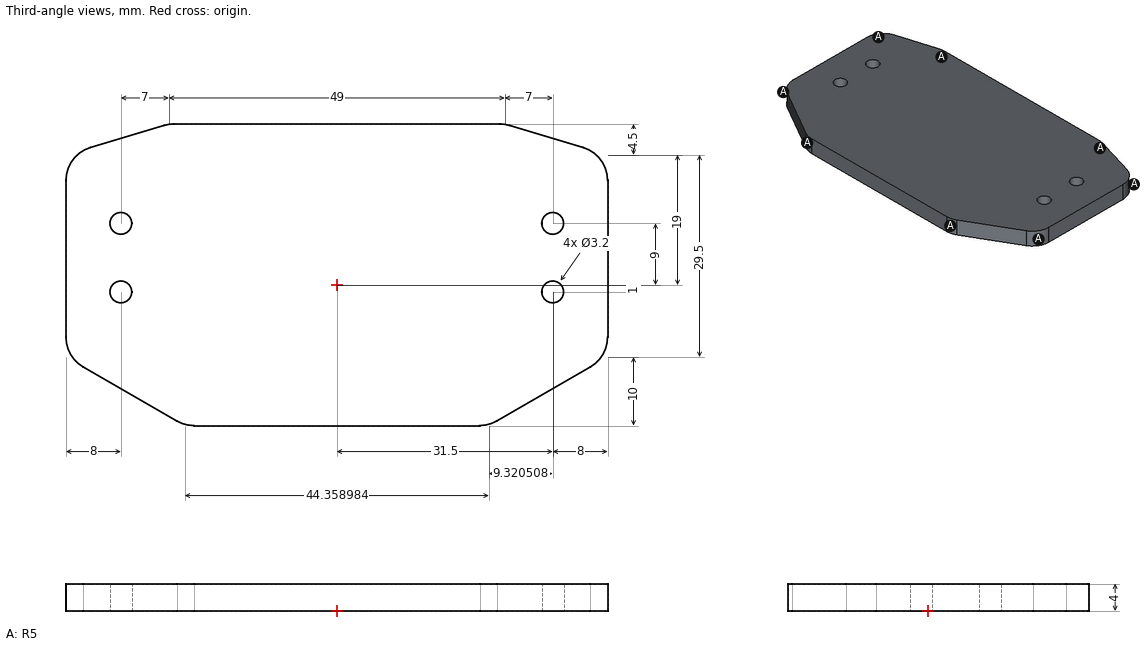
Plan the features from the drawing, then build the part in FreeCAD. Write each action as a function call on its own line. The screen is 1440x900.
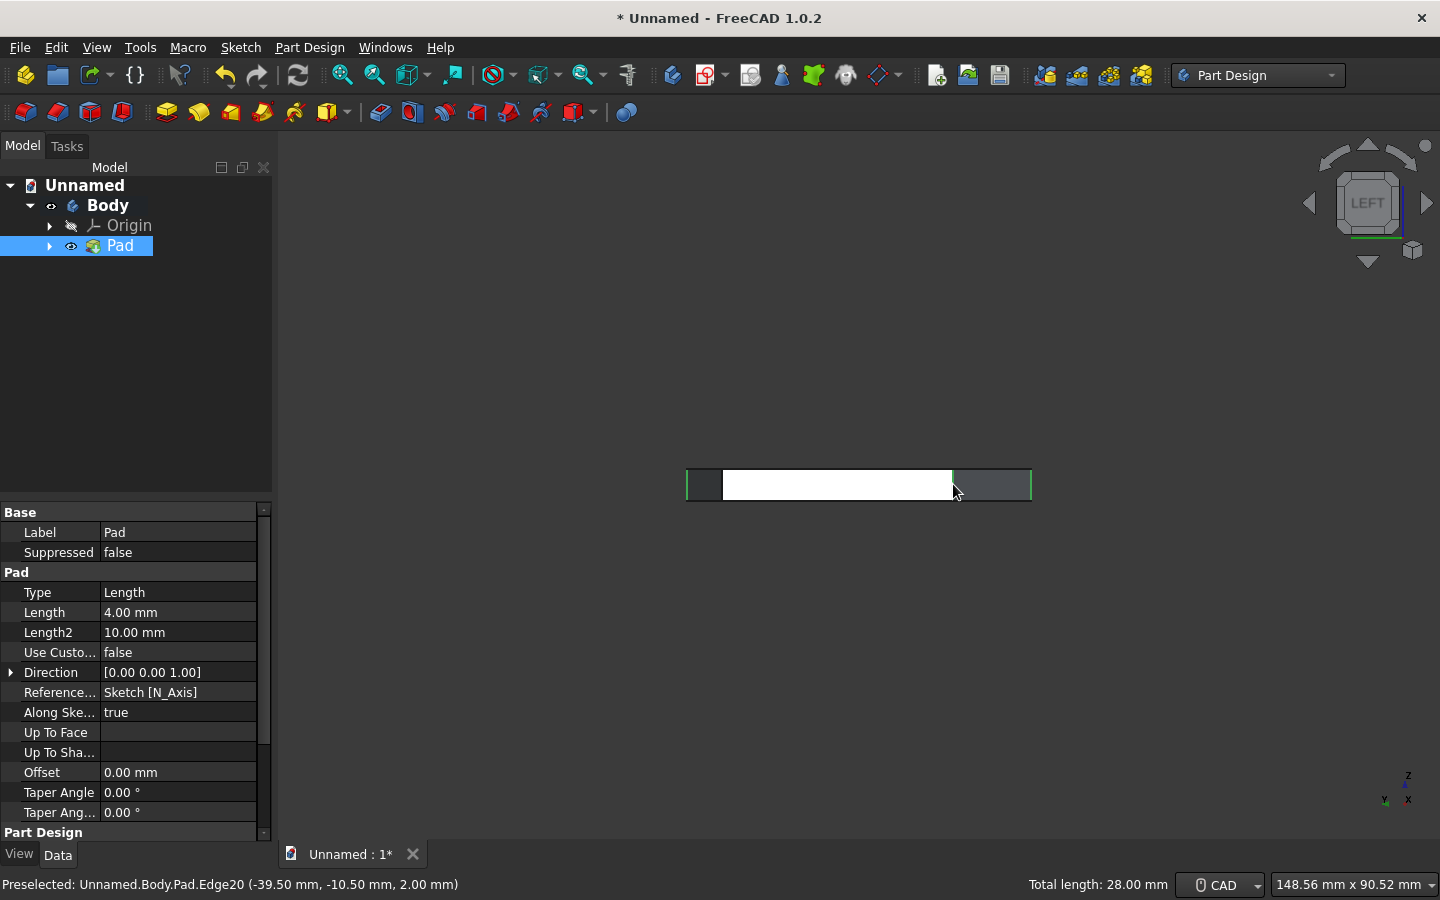
click(722, 484, ctrl)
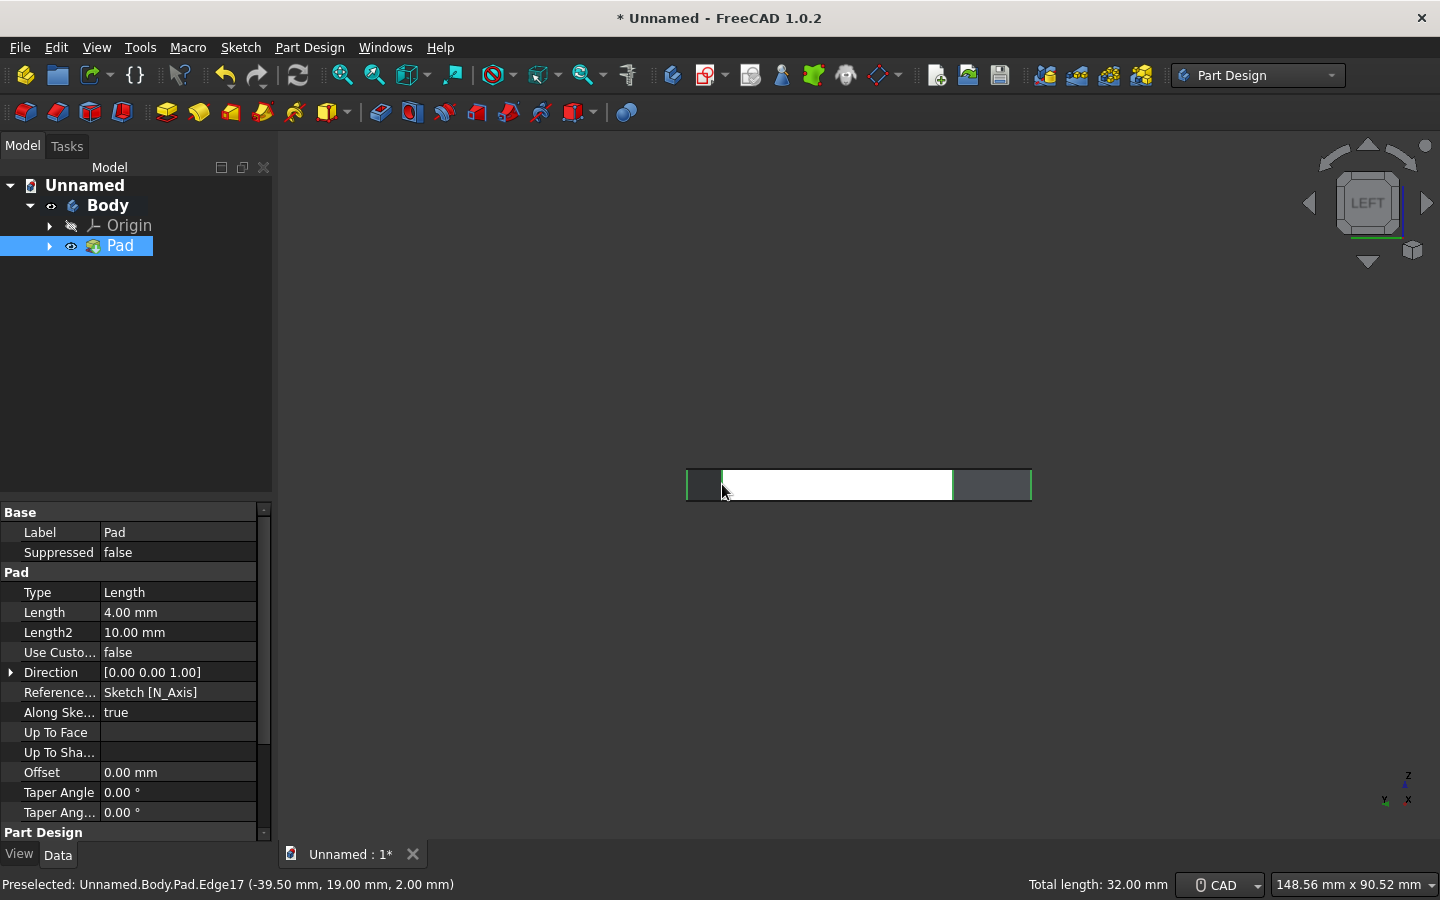
click(26, 112)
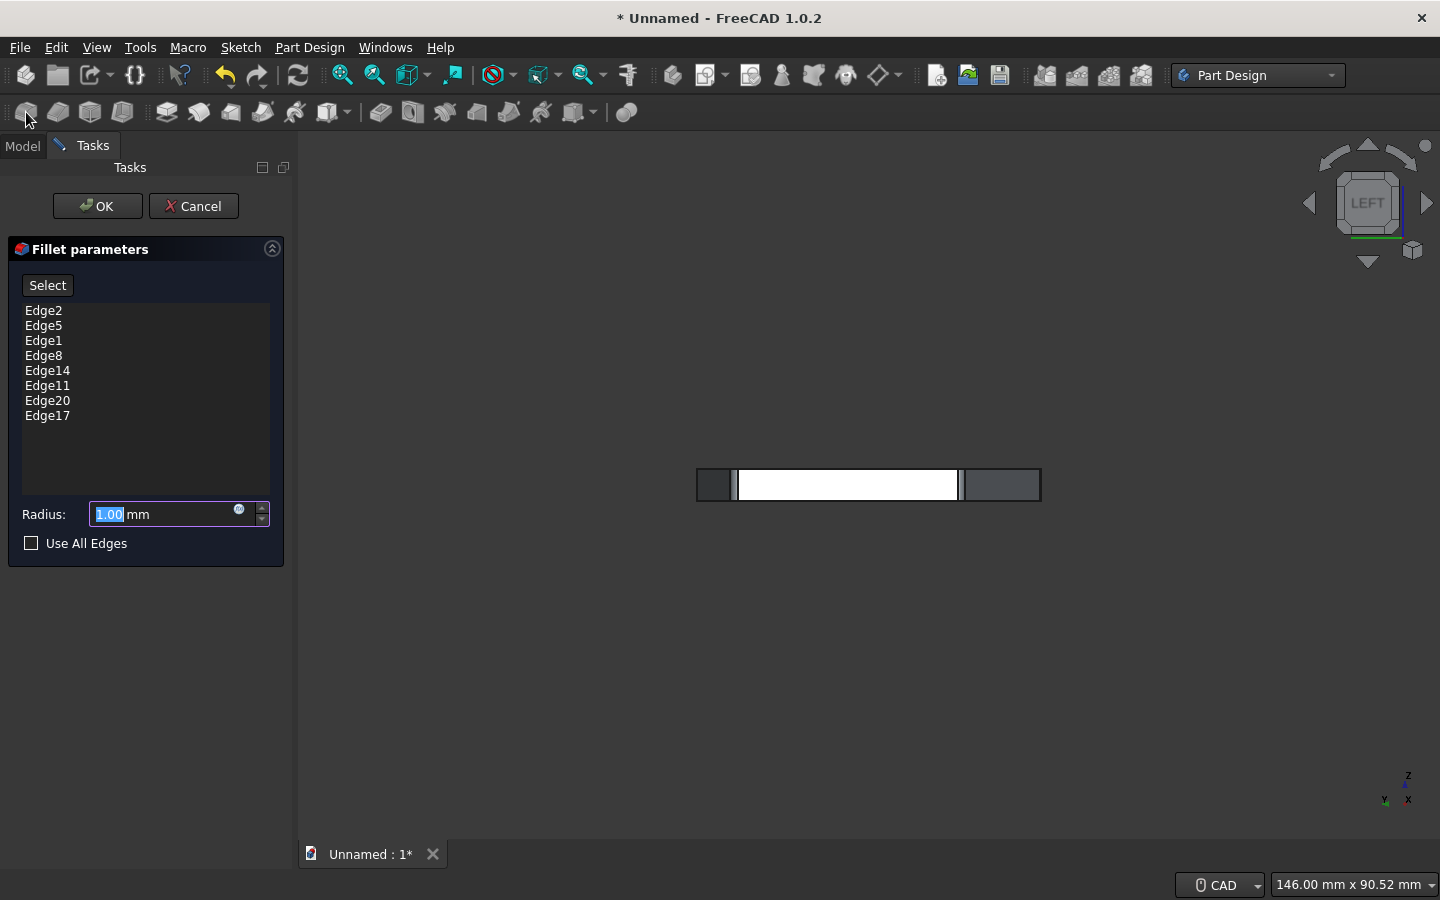
text(5)
key(Tab)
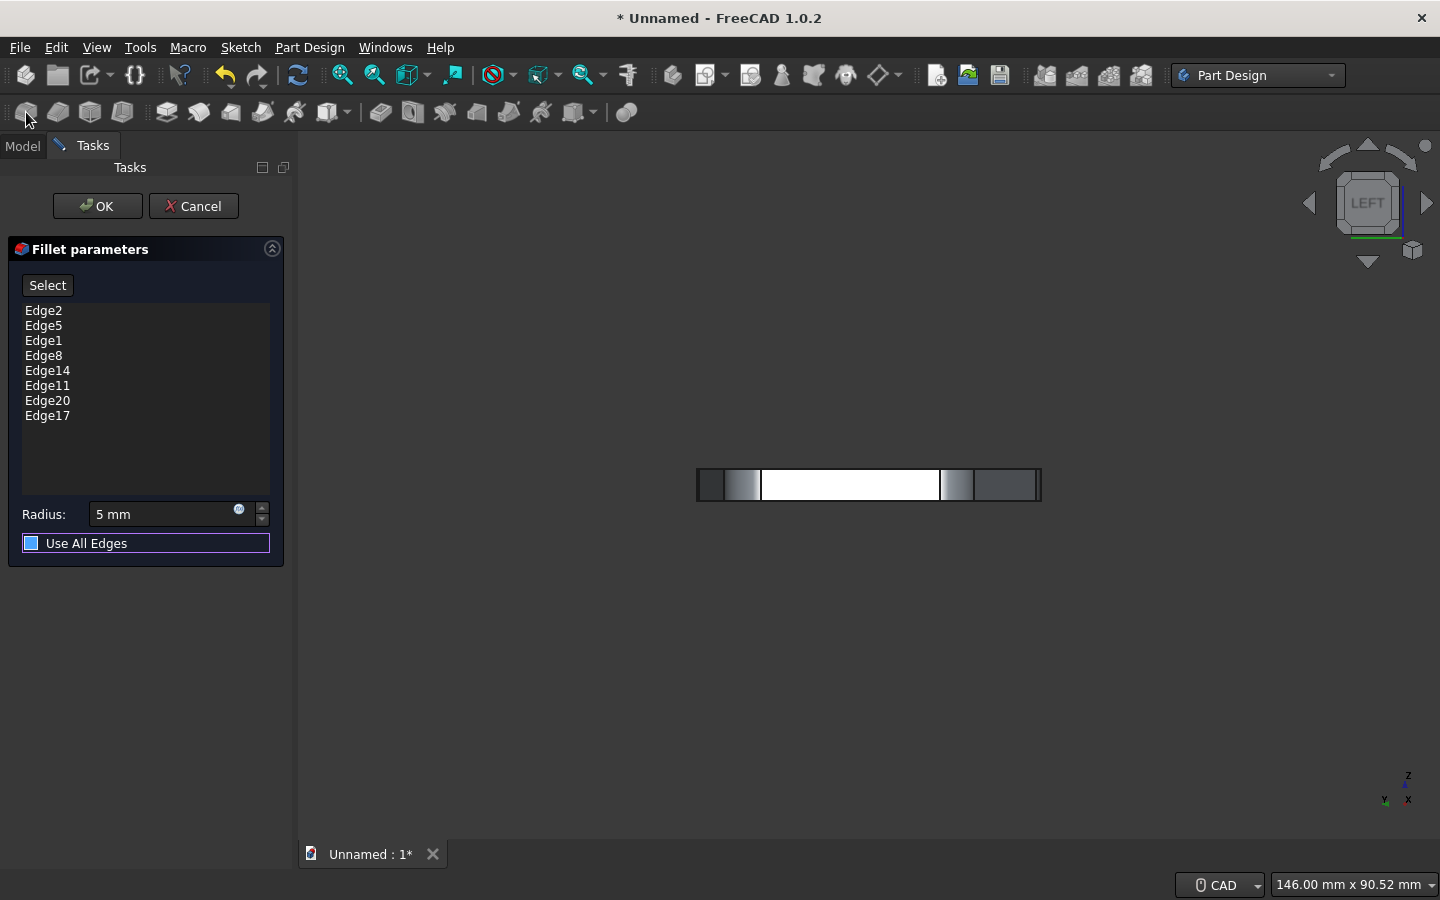
click(98, 206)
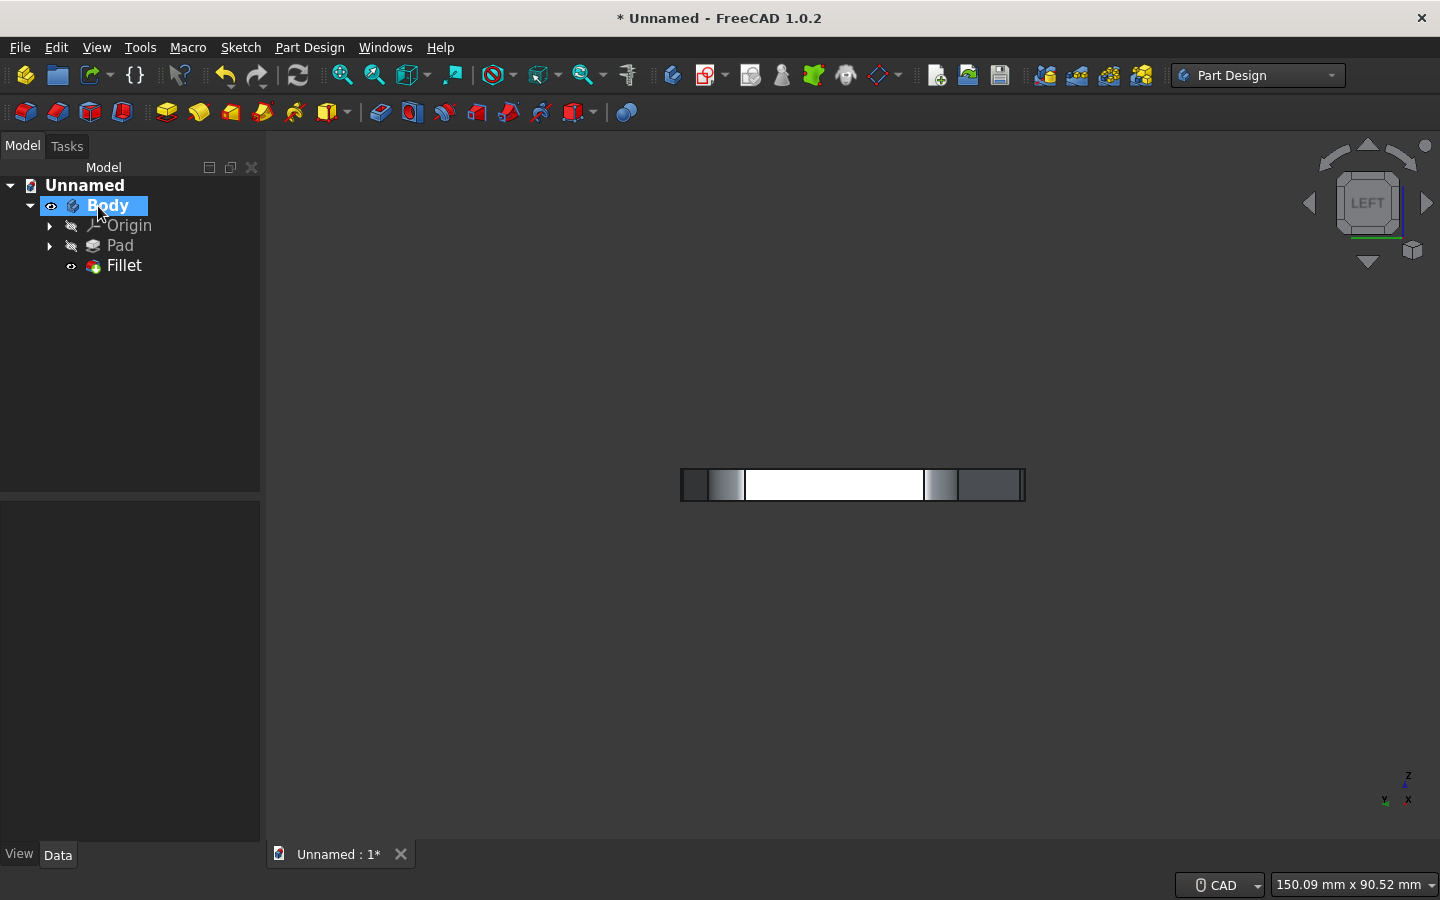
key(0)